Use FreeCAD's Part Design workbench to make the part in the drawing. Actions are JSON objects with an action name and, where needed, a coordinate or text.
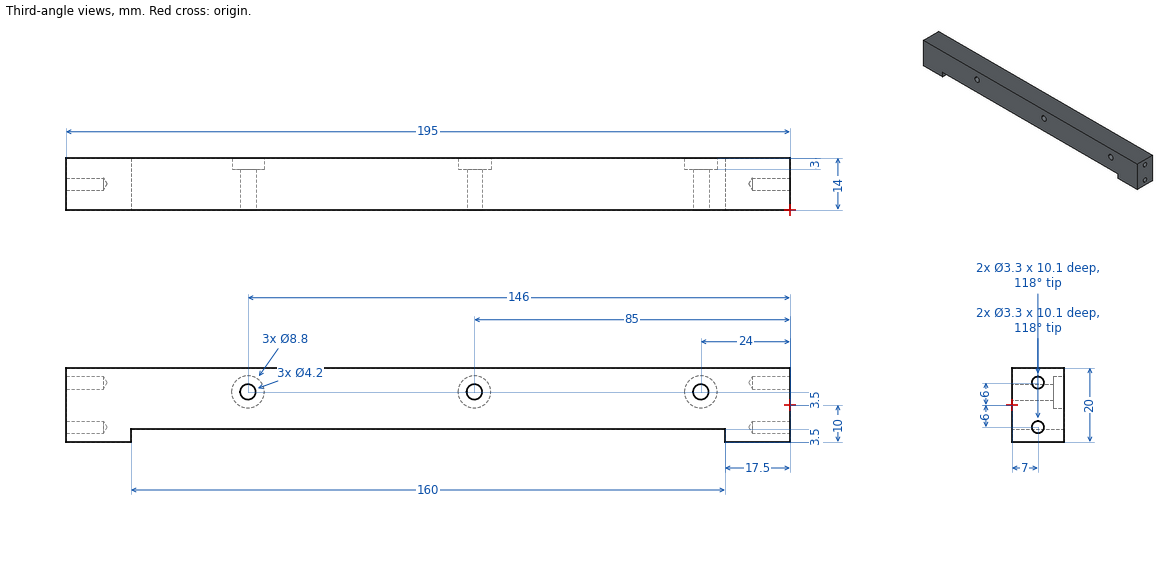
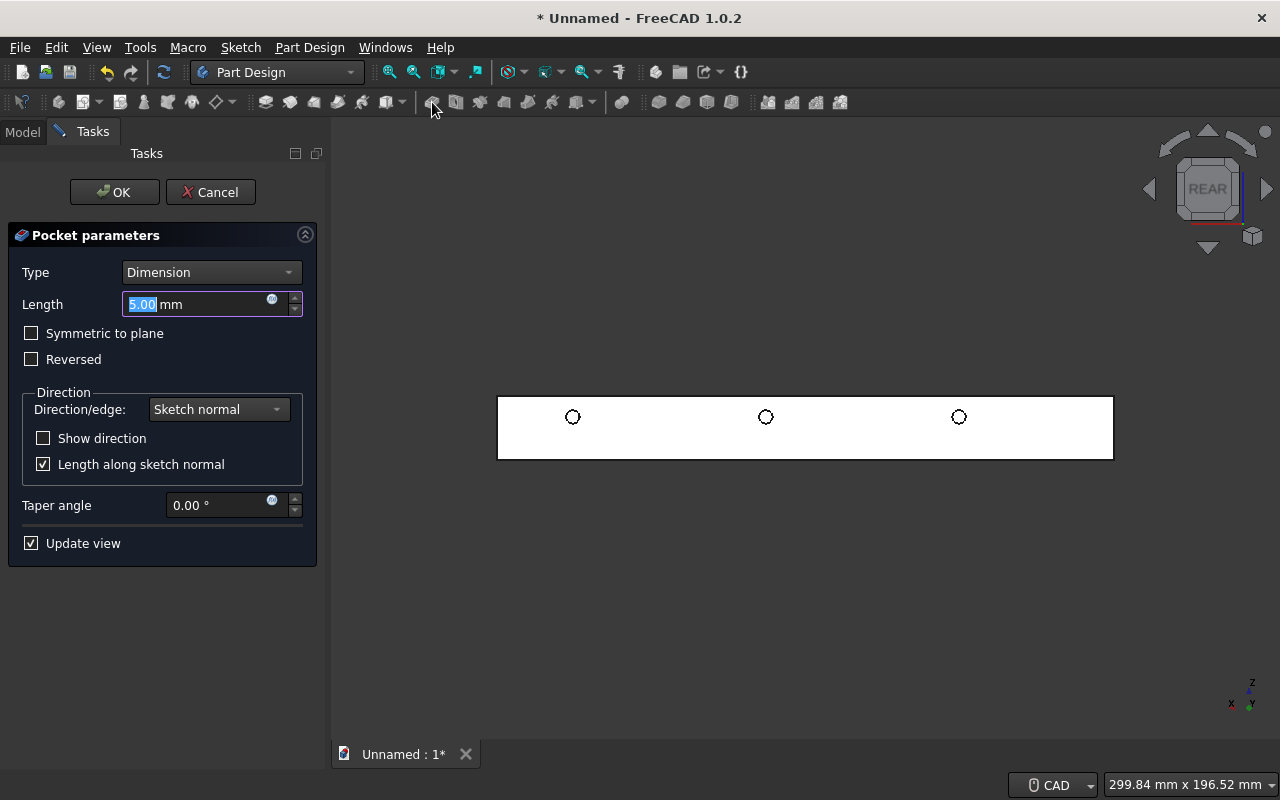
{"action": "left_click", "coordinate": [212, 272]}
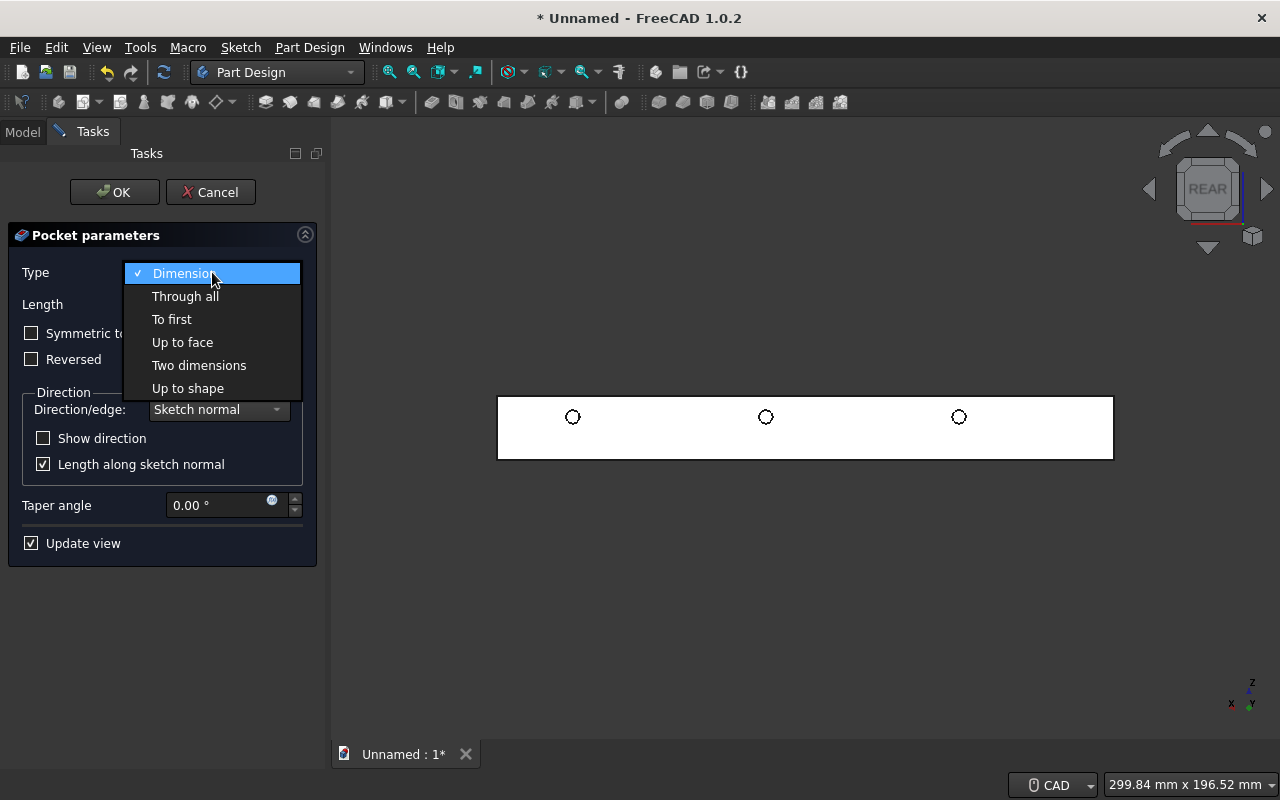
{"action": "left_click", "coordinate": [212, 296]}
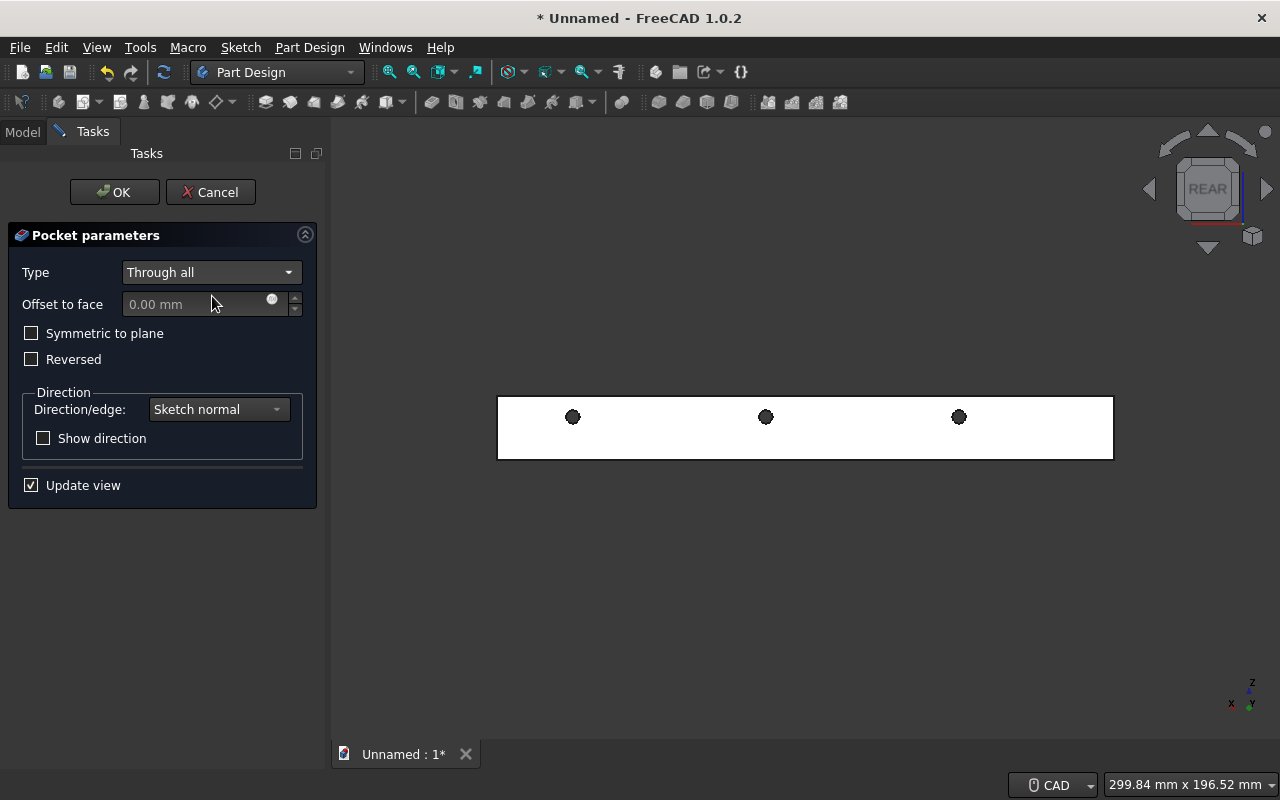
{"action": "left_click", "coordinate": [115, 192]}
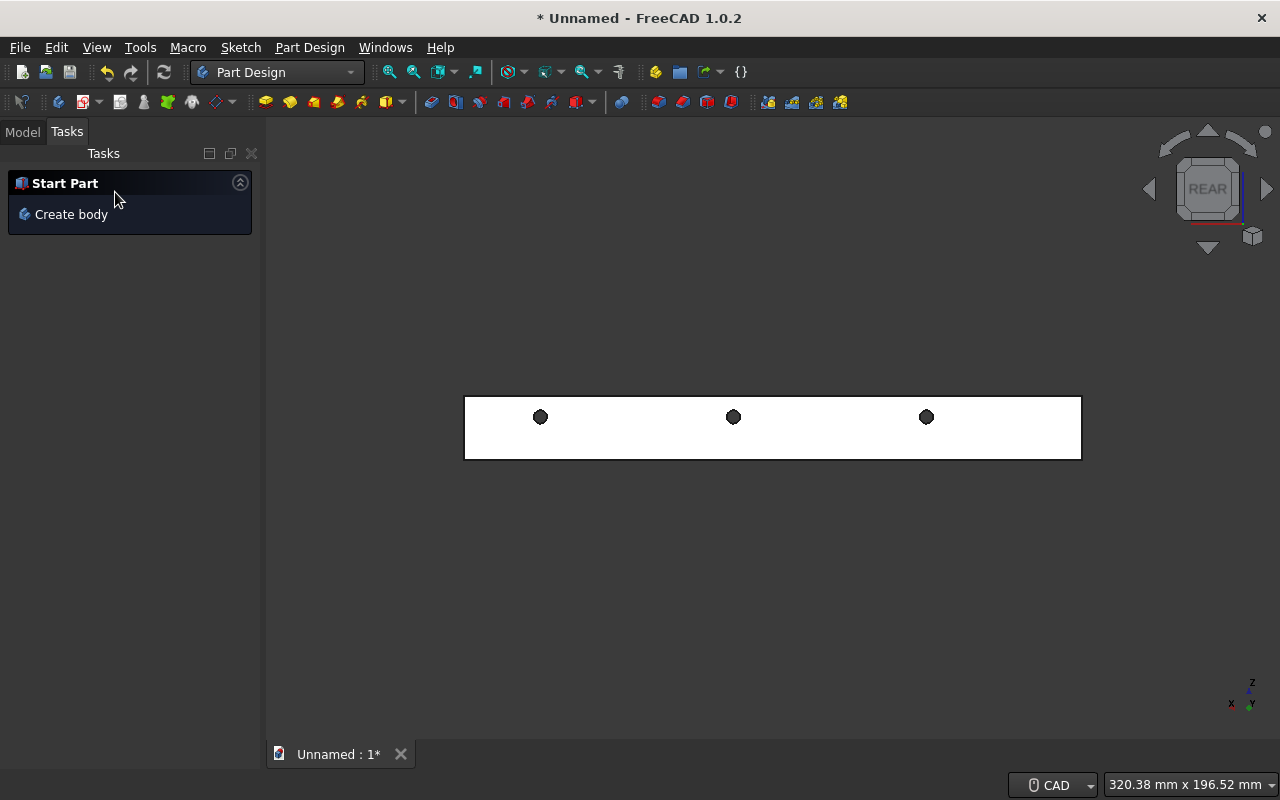
{"action": "left_click", "coordinate": [597, 427]}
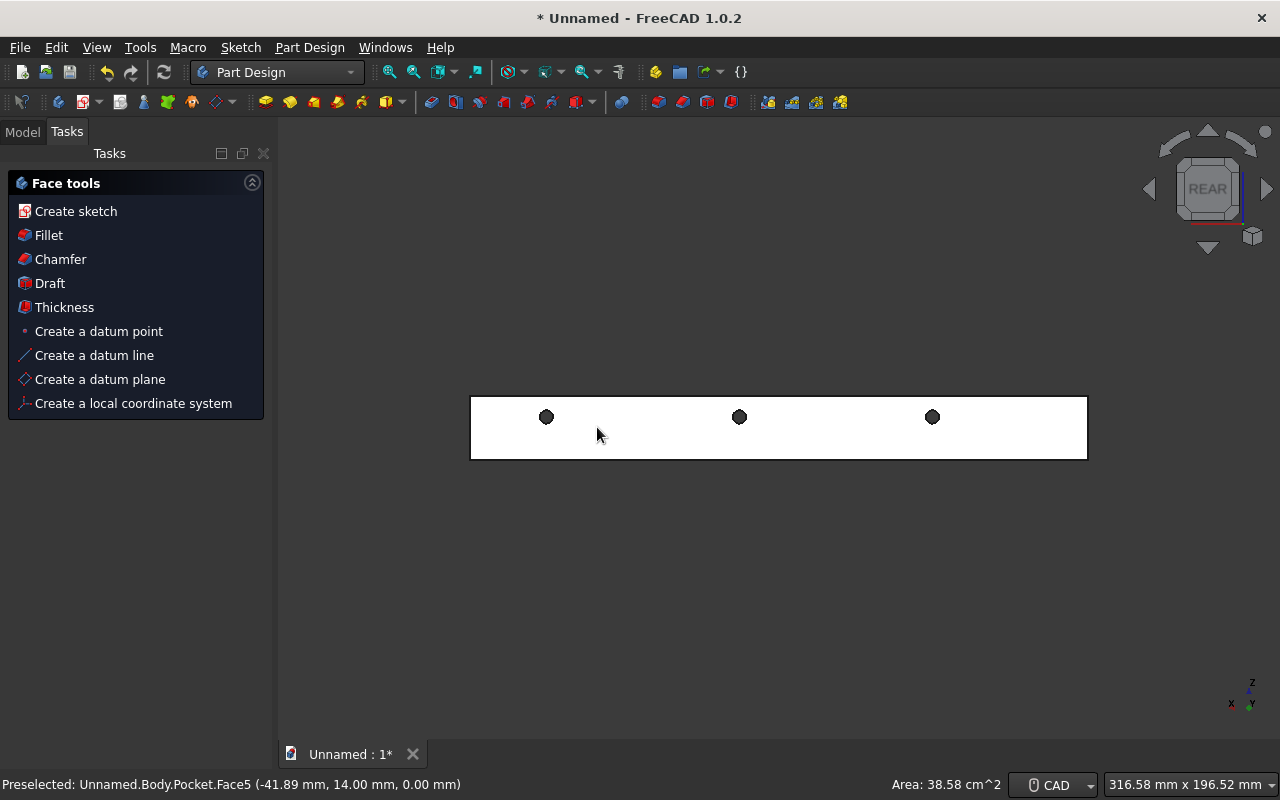
{"action": "left_click", "coordinate": [84, 102]}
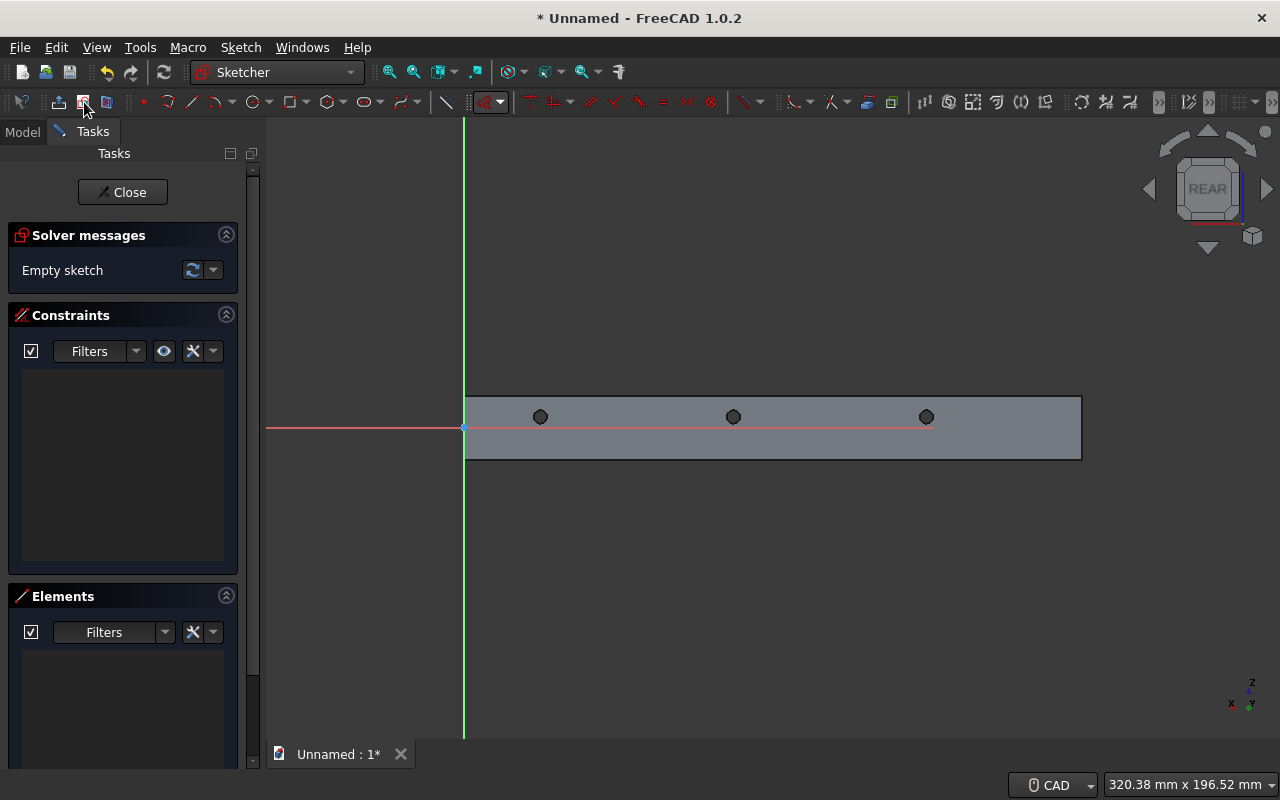
{"action": "key", "text": "g c"}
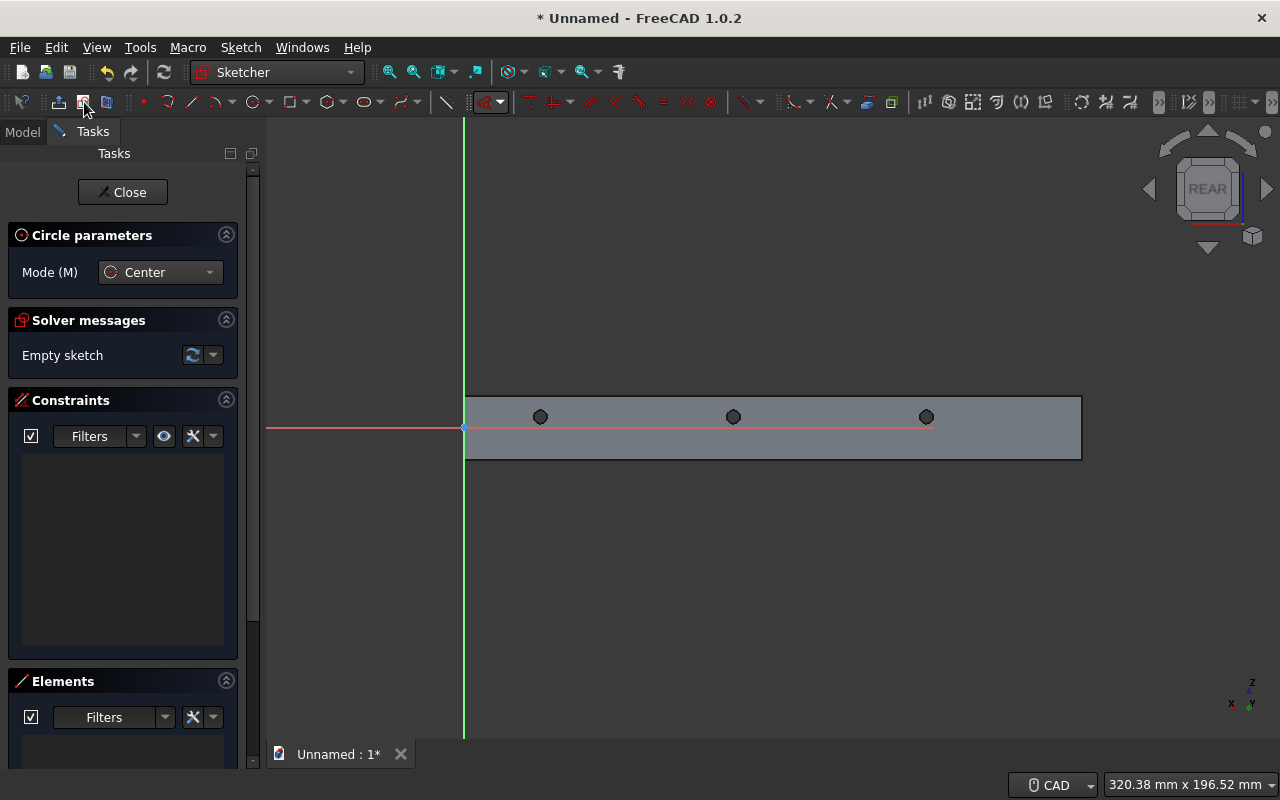
{"action": "scroll", "coordinate": [927, 417], "scroll_direction": "up", "scroll_amount": 3}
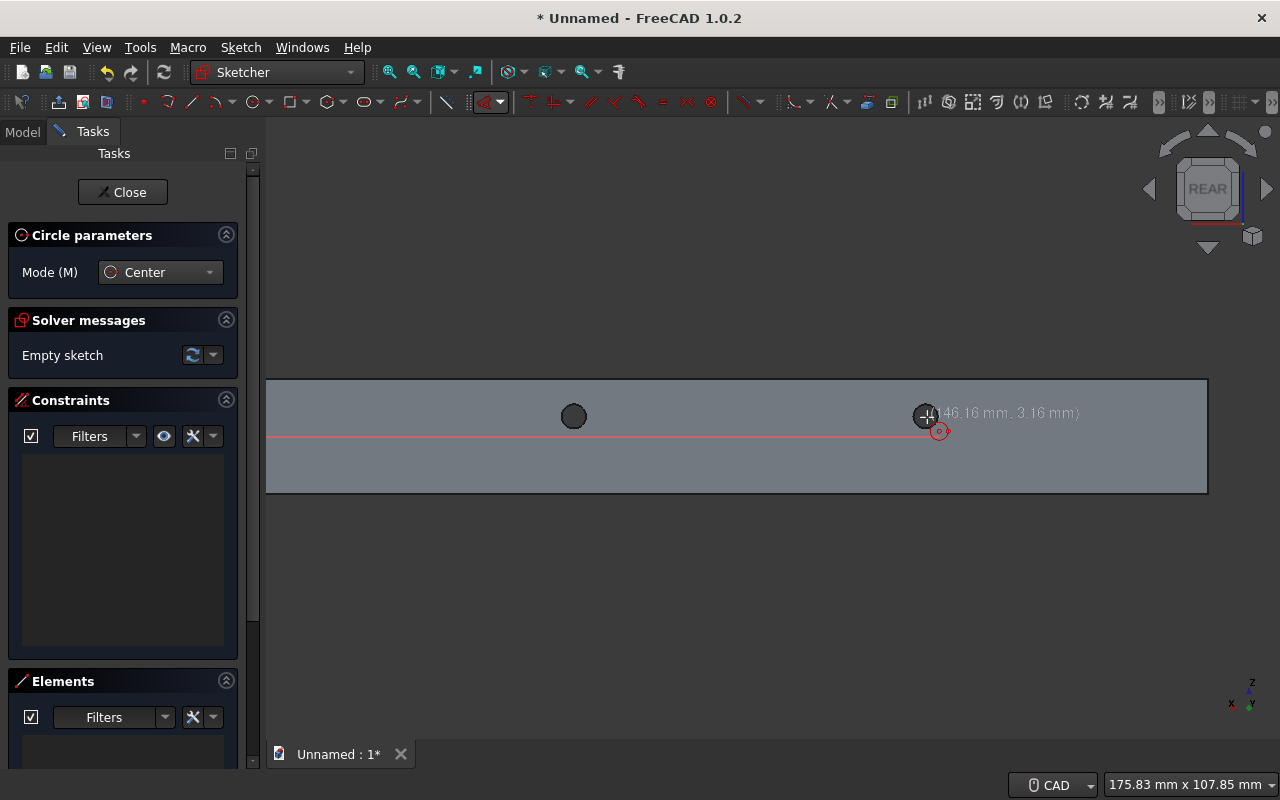
{"action": "left_click", "coordinate": [926, 416]}
{"action": "left_click", "coordinate": [944, 399]}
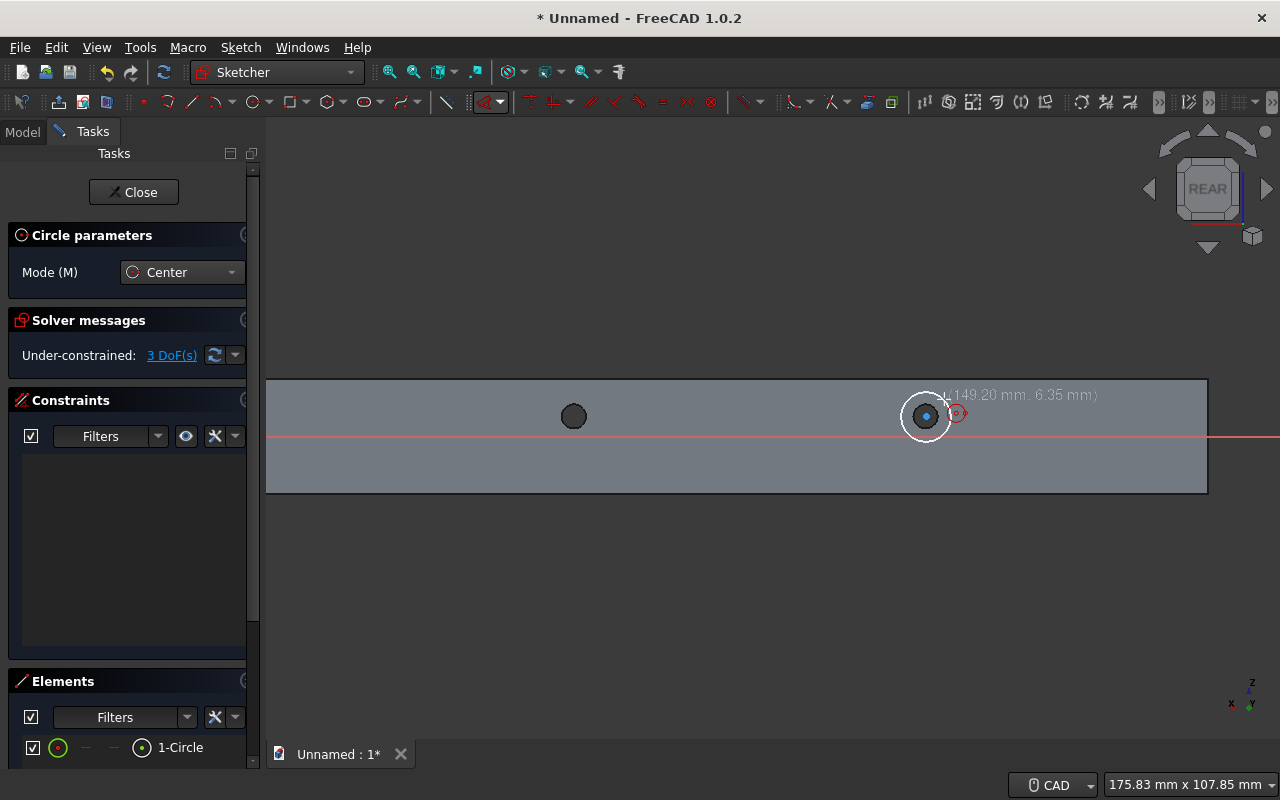
{"action": "left_click", "coordinate": [574, 416]}
{"action": "left_click", "coordinate": [592, 399]}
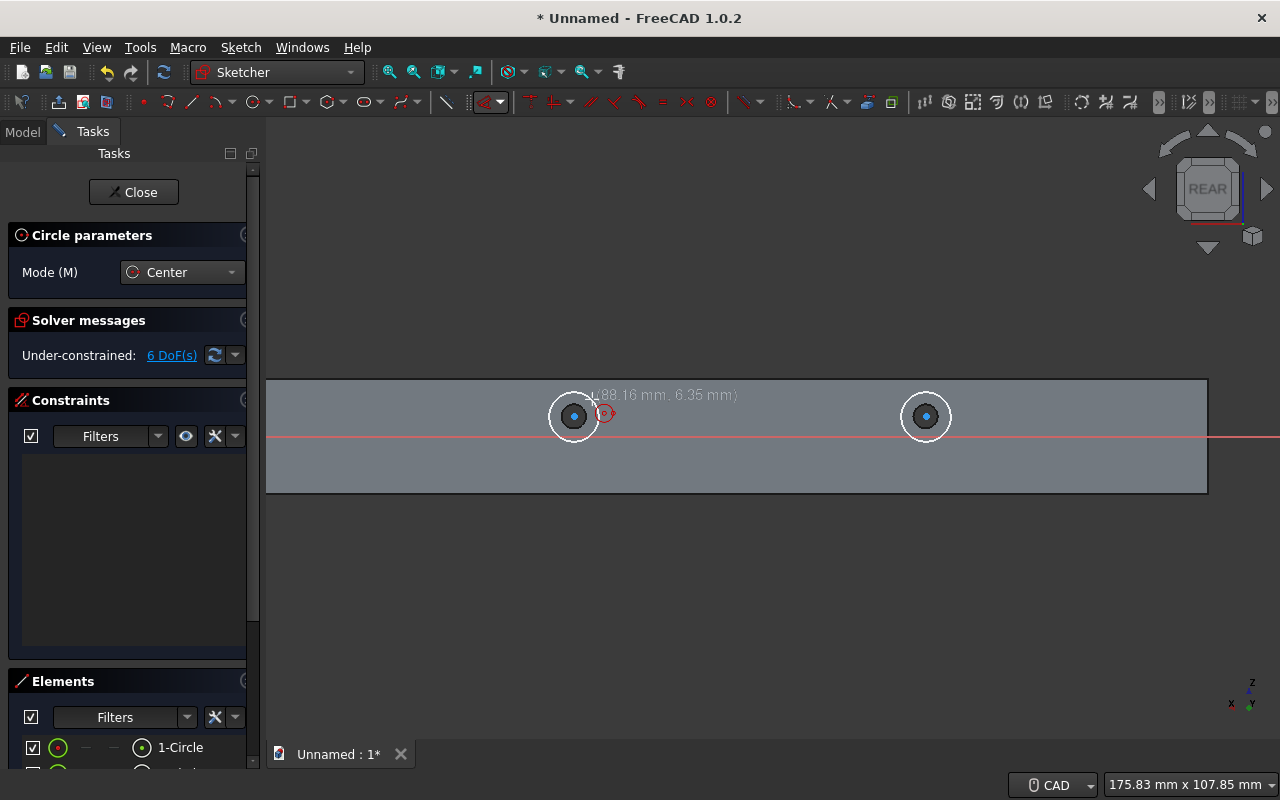
{"action": "scroll", "coordinate": [1085, 451], "scroll_direction": "down", "scroll_amount": 2}